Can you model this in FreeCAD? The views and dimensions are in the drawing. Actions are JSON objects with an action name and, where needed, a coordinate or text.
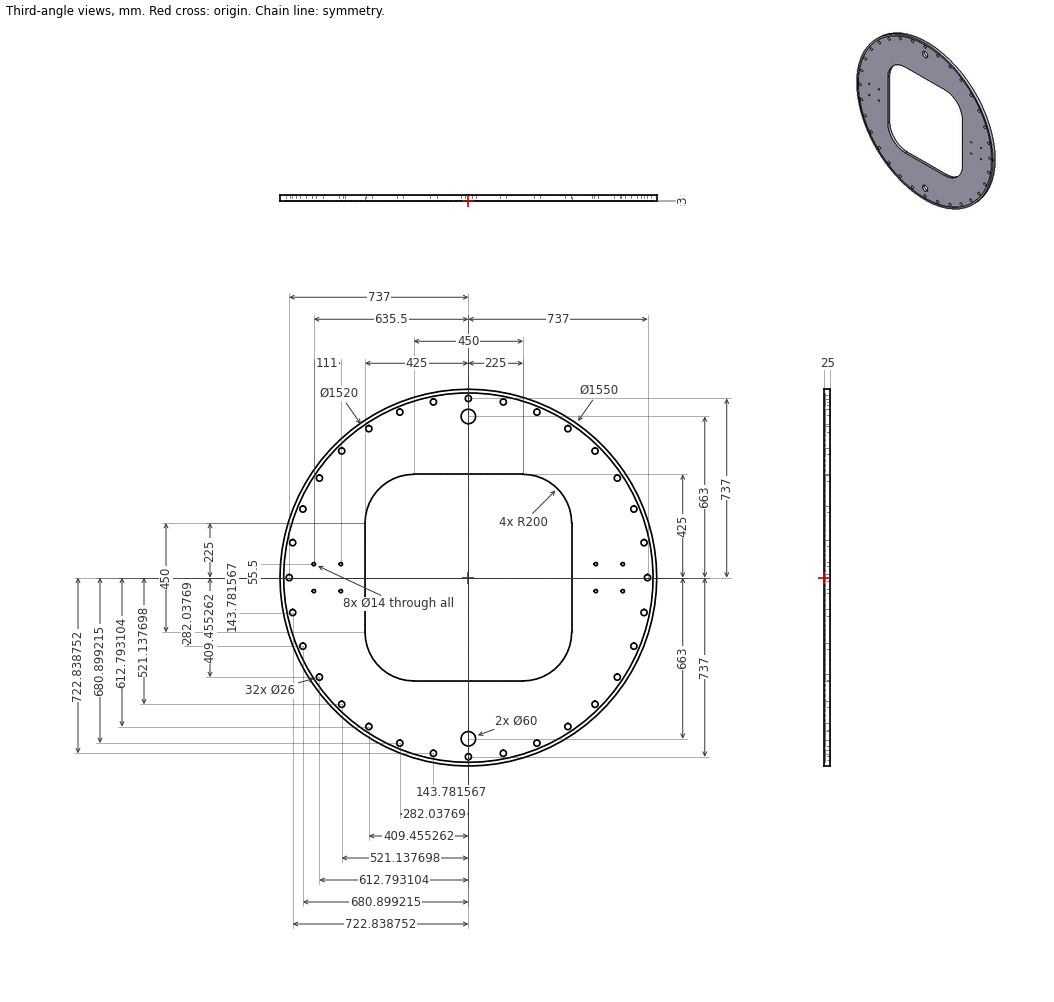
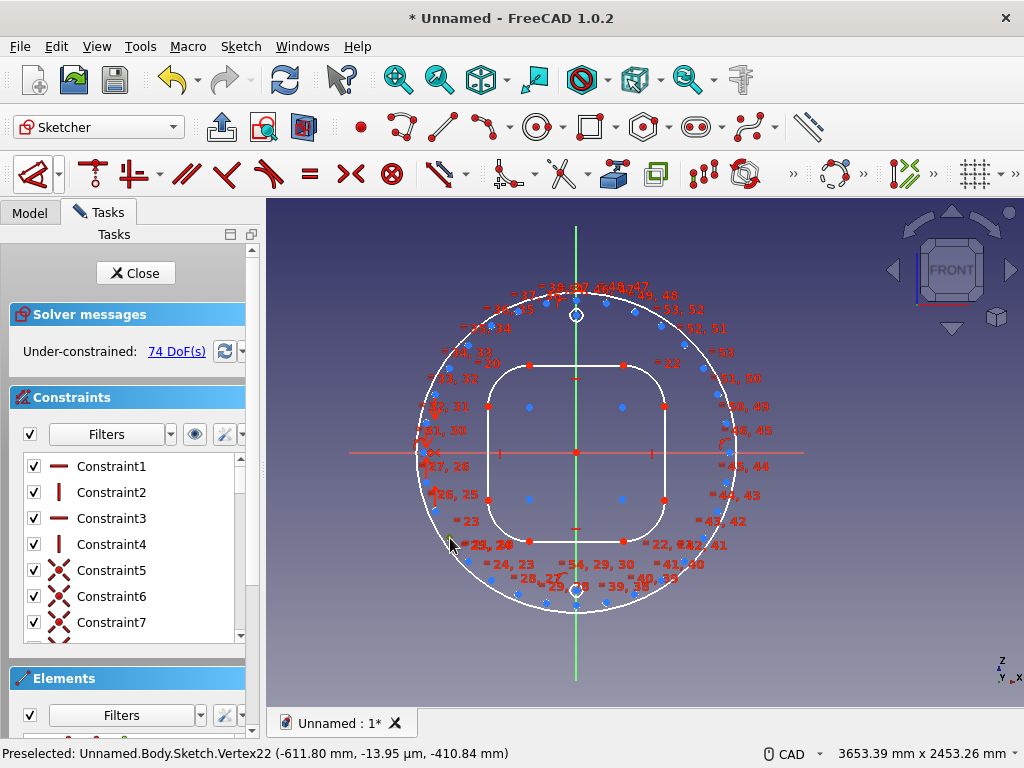
{"action": "left_click", "coordinate": [449, 368]}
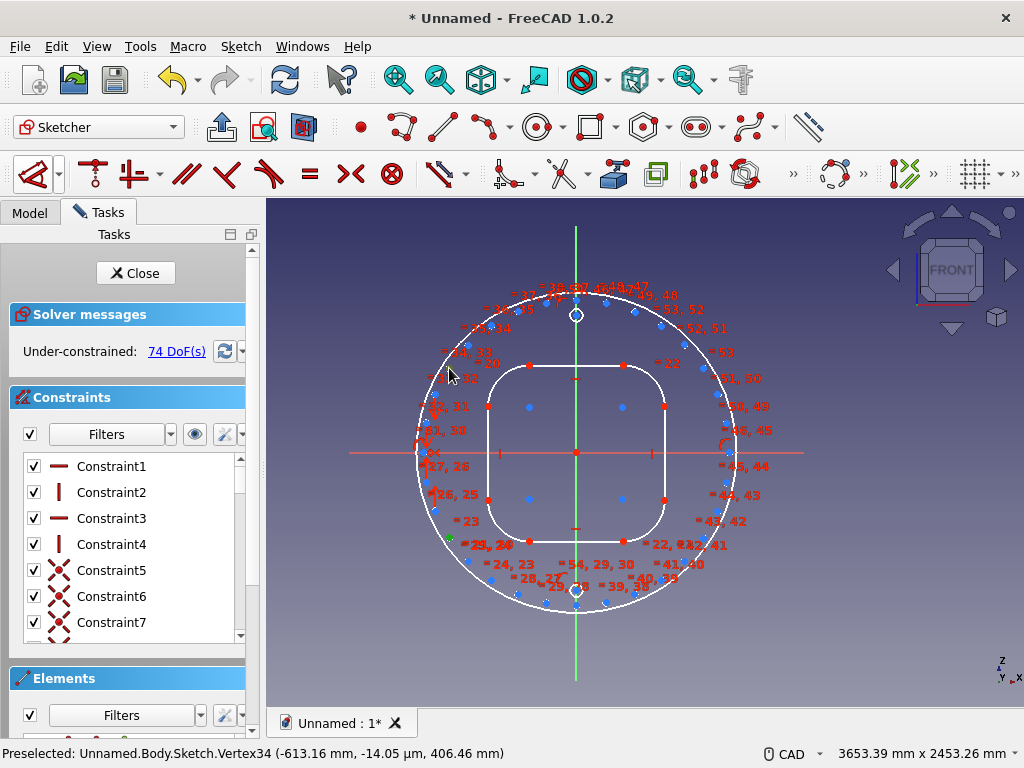
{"action": "left_click", "coordinate": [375, 453]}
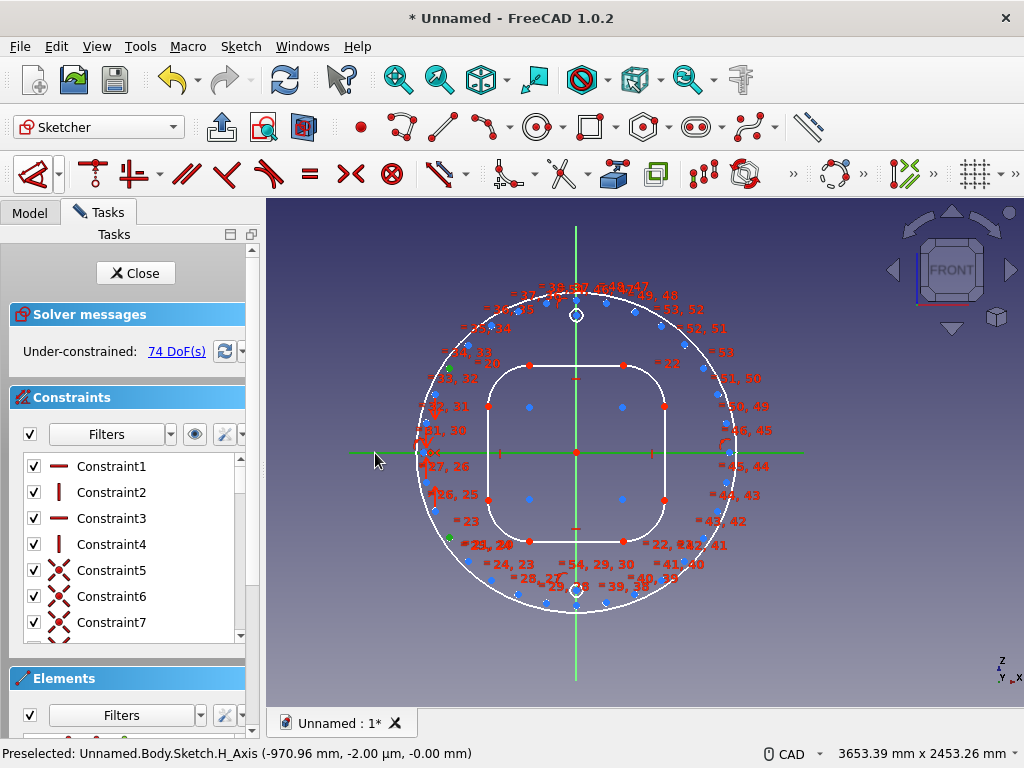
{"action": "left_click", "coordinate": [351, 174]}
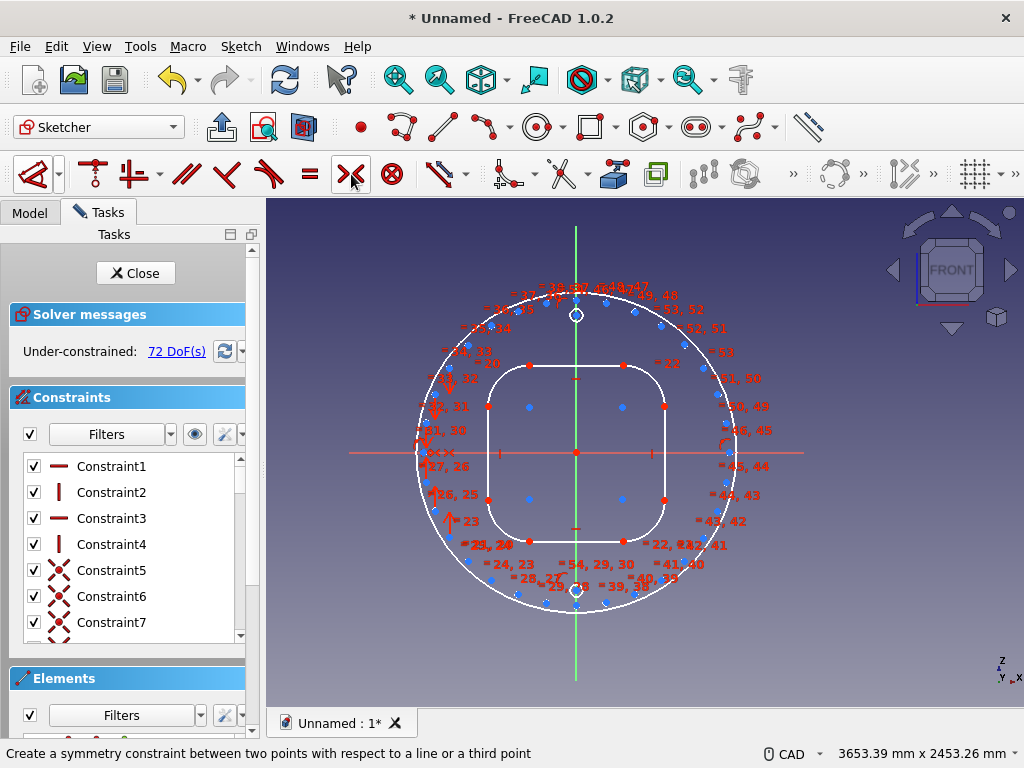
{"action": "left_click", "coordinate": [468, 561]}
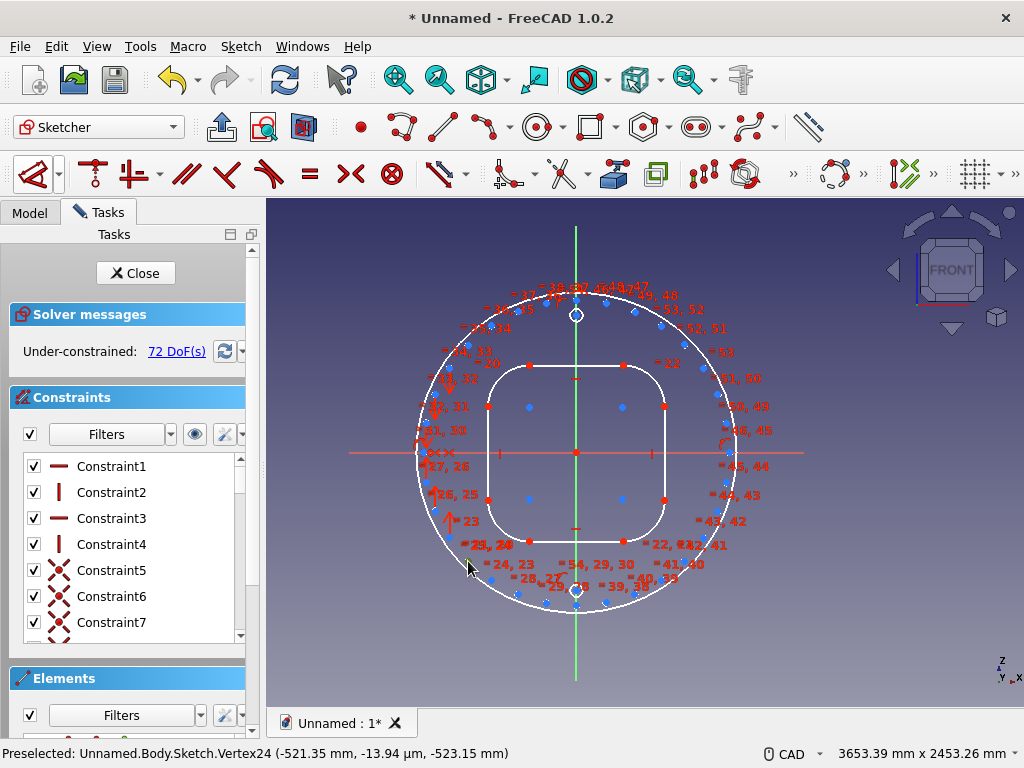
{"action": "left_click", "coordinate": [468, 345]}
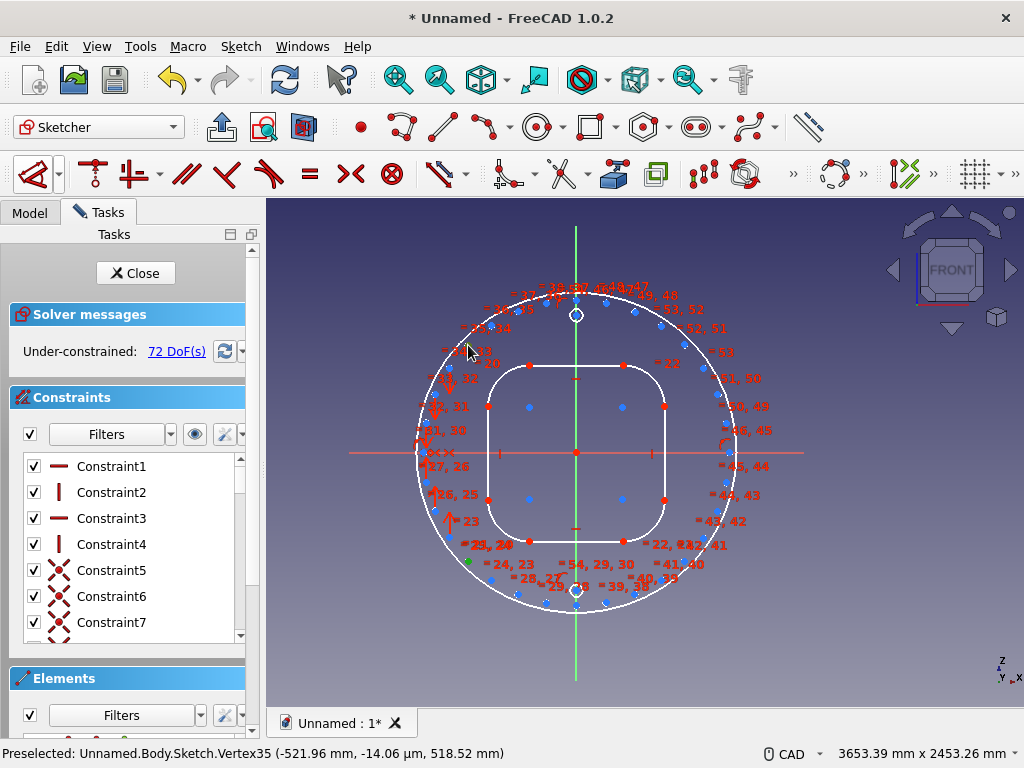
{"action": "left_click", "coordinate": [375, 453]}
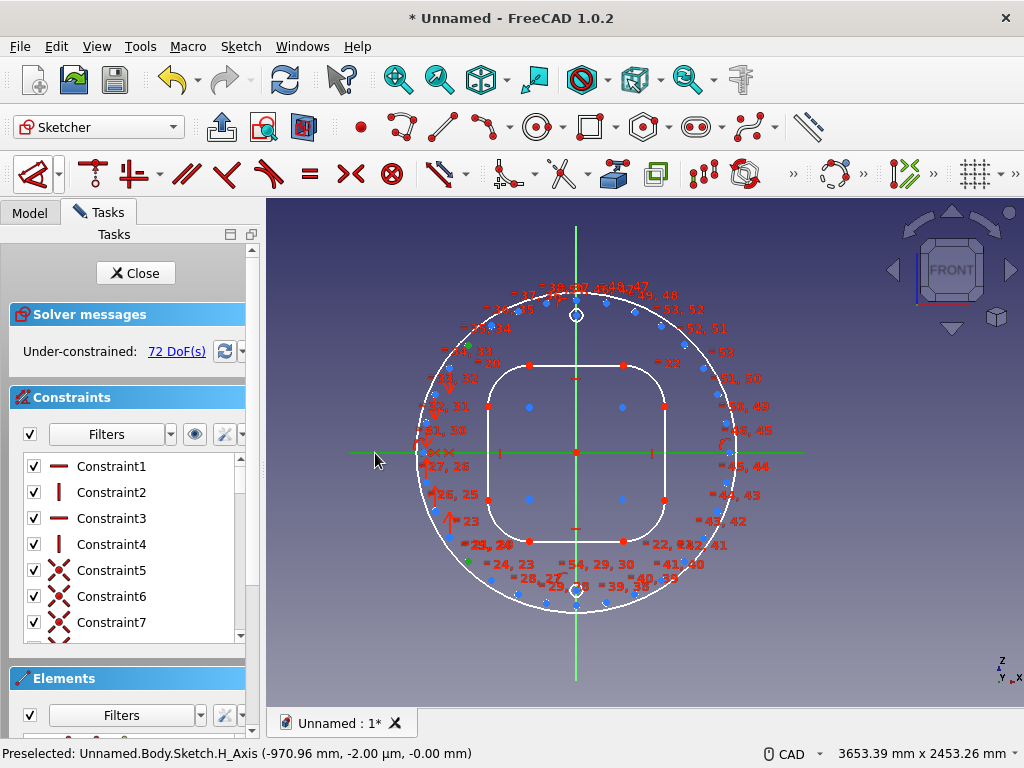
{"action": "left_click", "coordinate": [351, 174]}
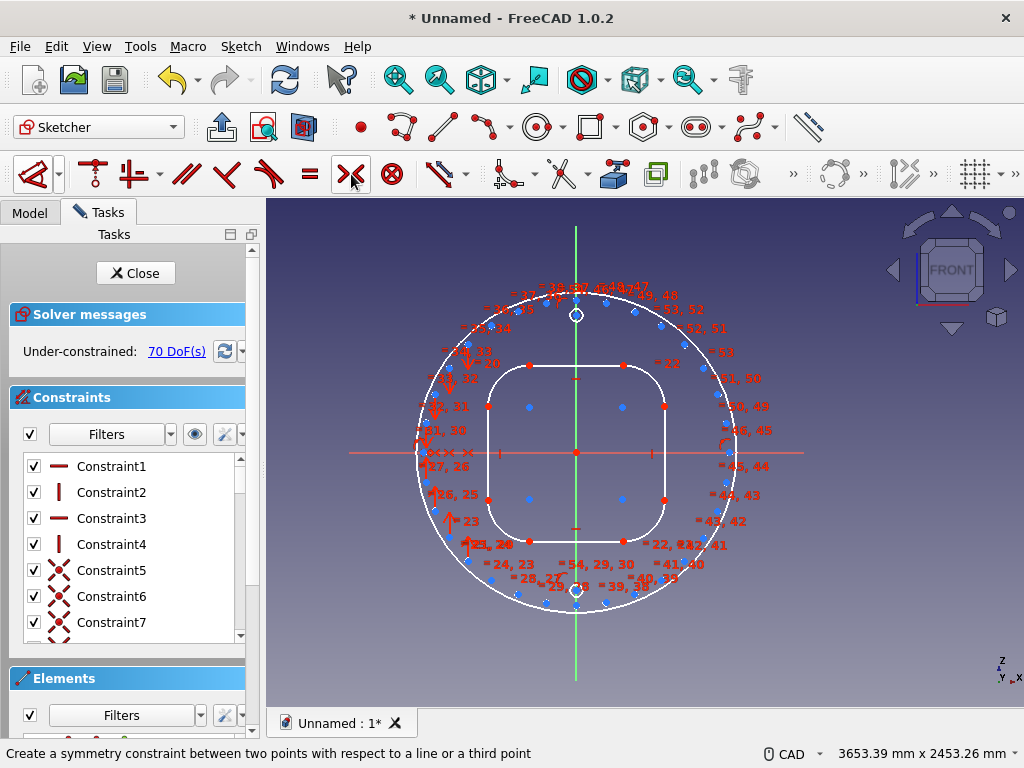
{"action": "left_click", "coordinate": [491, 581]}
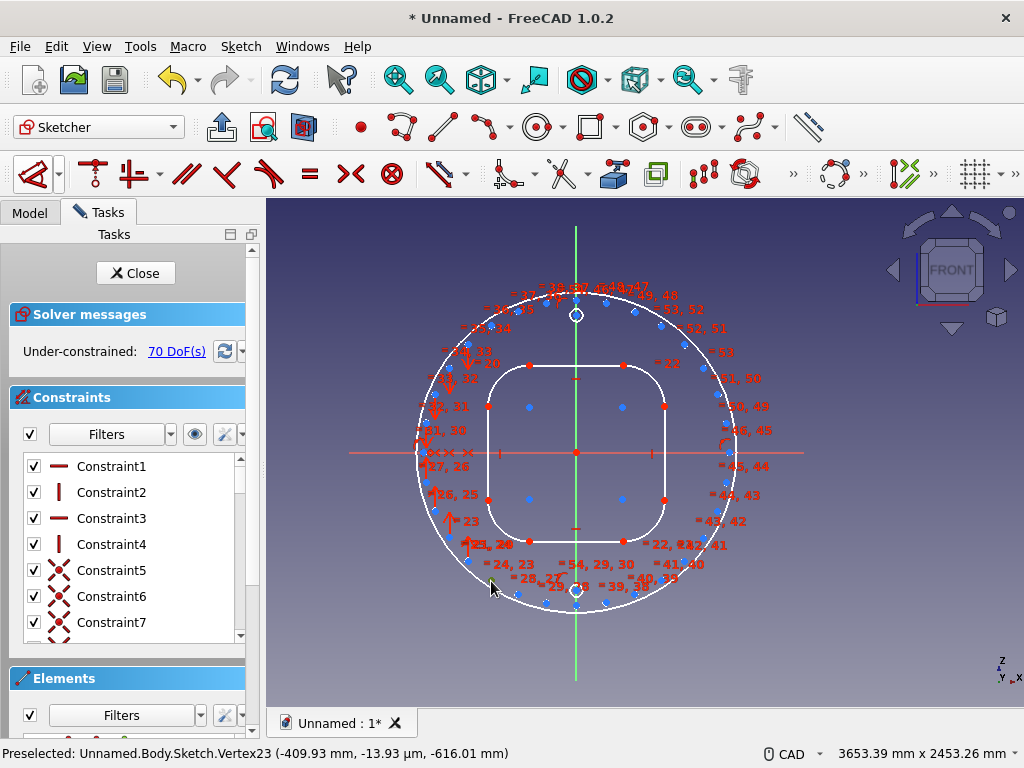
{"action": "left_click", "coordinate": [491, 326]}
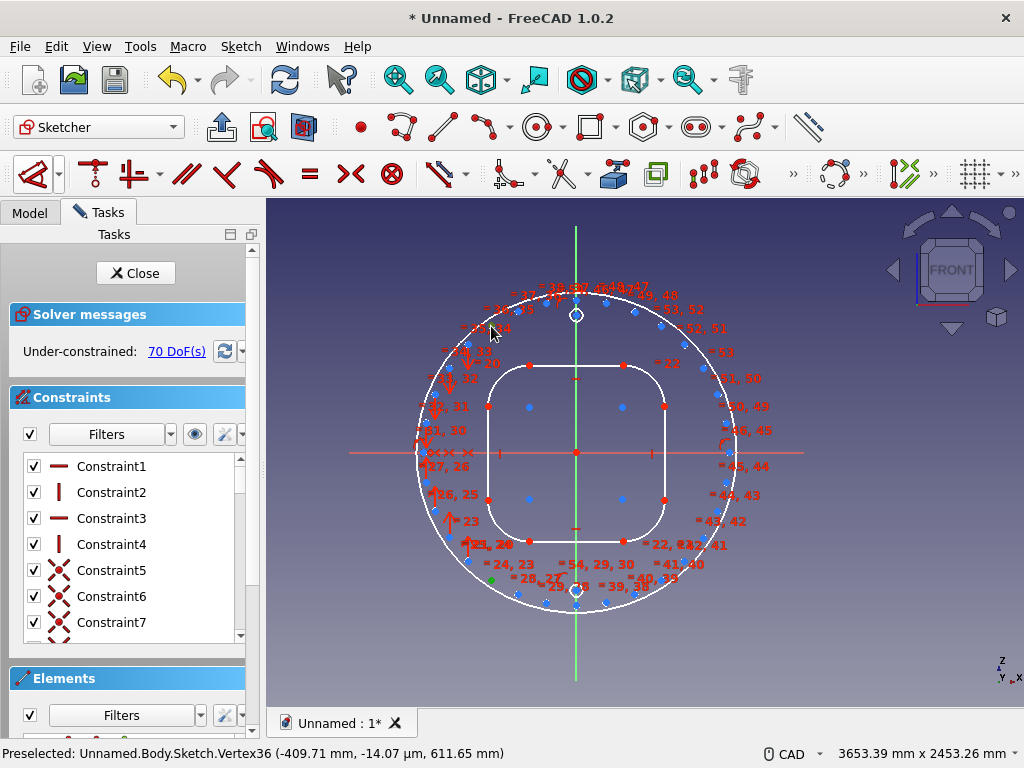
{"action": "left_click", "coordinate": [375, 453]}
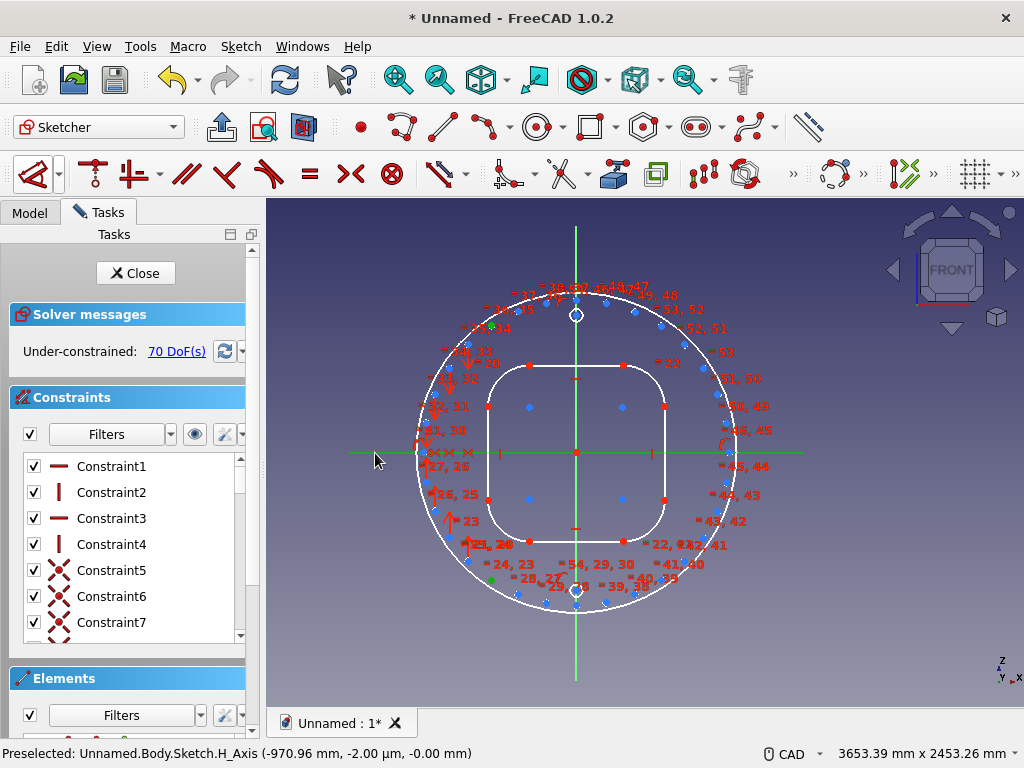
{"action": "left_click", "coordinate": [351, 174]}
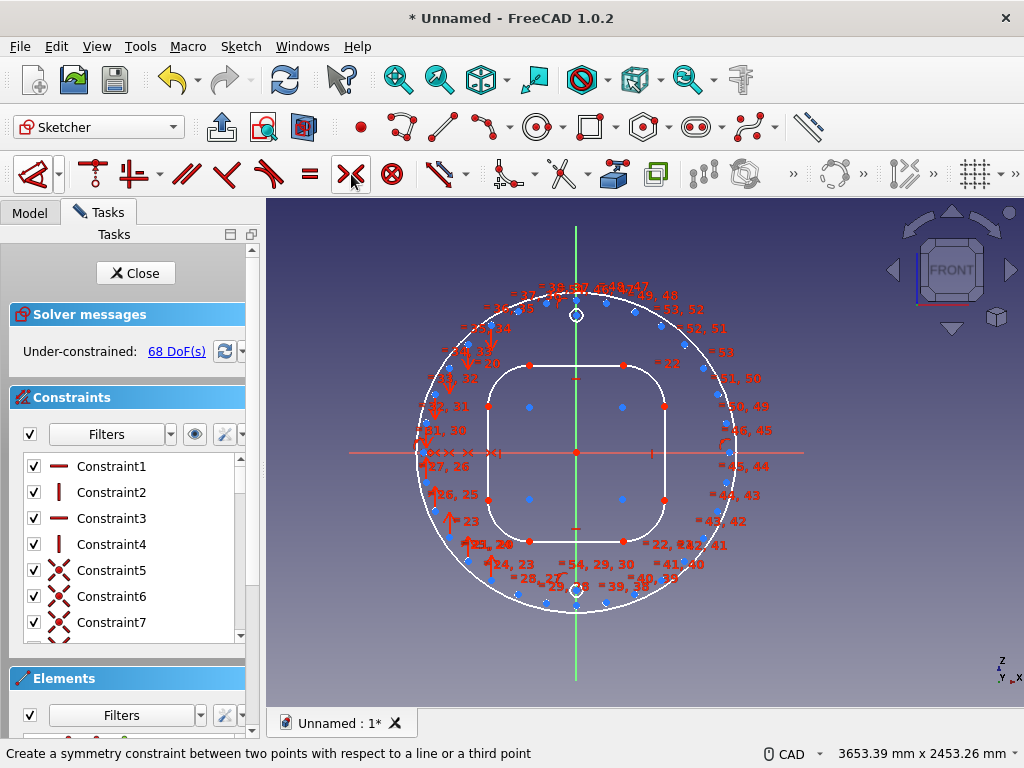
{"action": "left_click", "coordinate": [518, 595]}